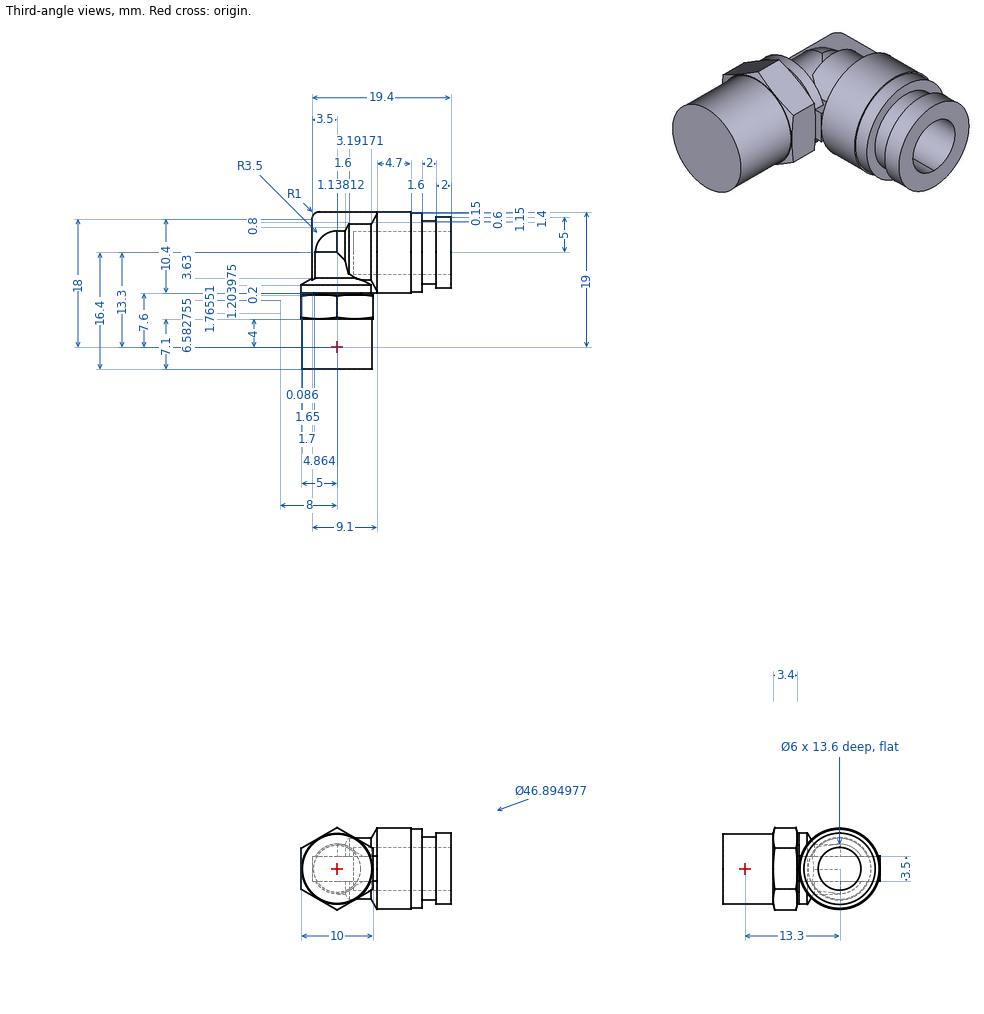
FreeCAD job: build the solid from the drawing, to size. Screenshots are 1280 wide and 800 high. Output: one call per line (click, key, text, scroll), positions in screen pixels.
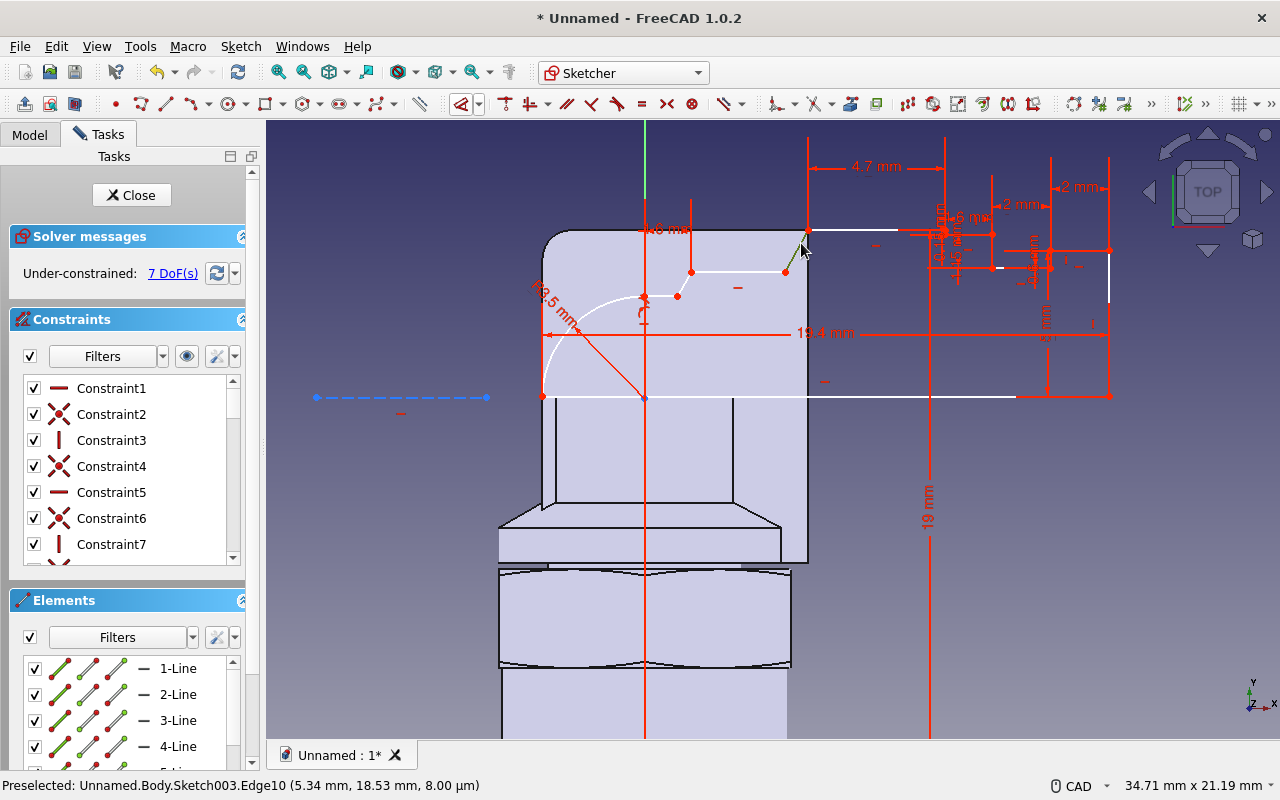
key(i)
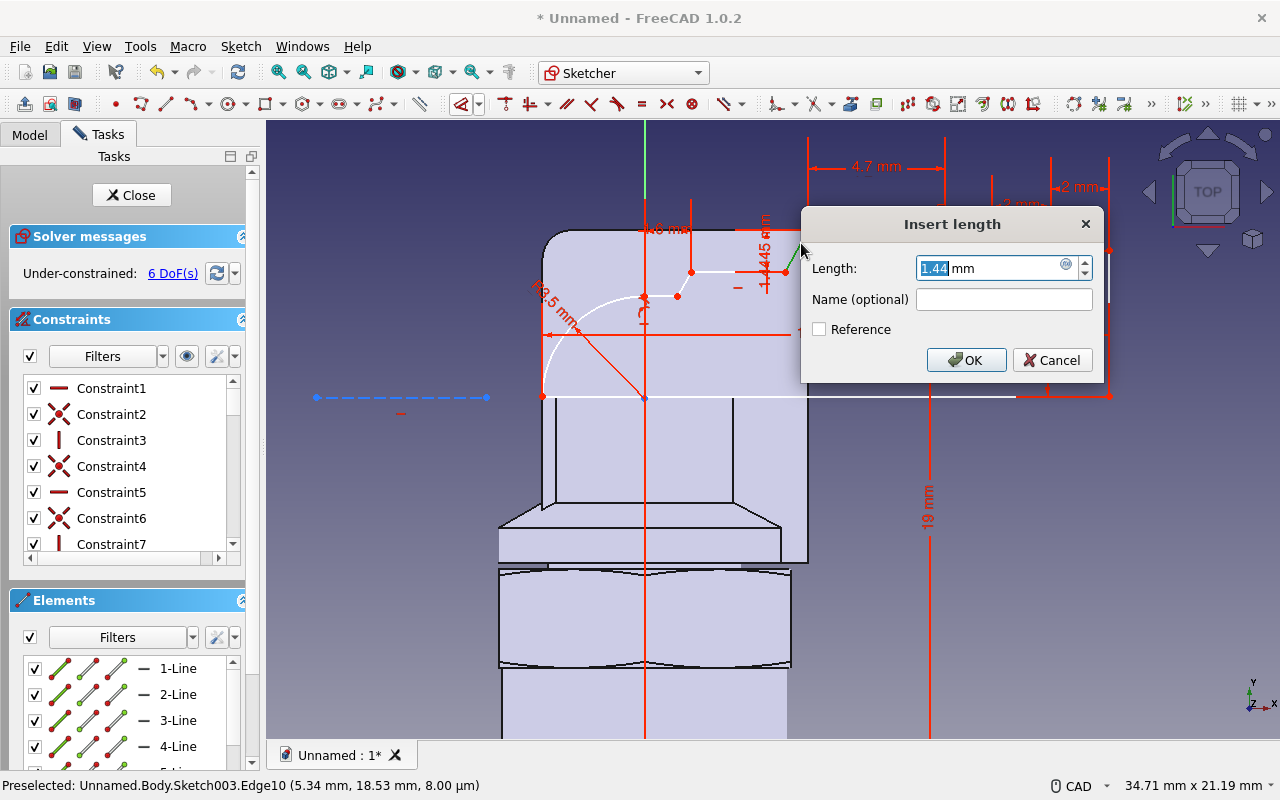
text(1.4)
key(Return)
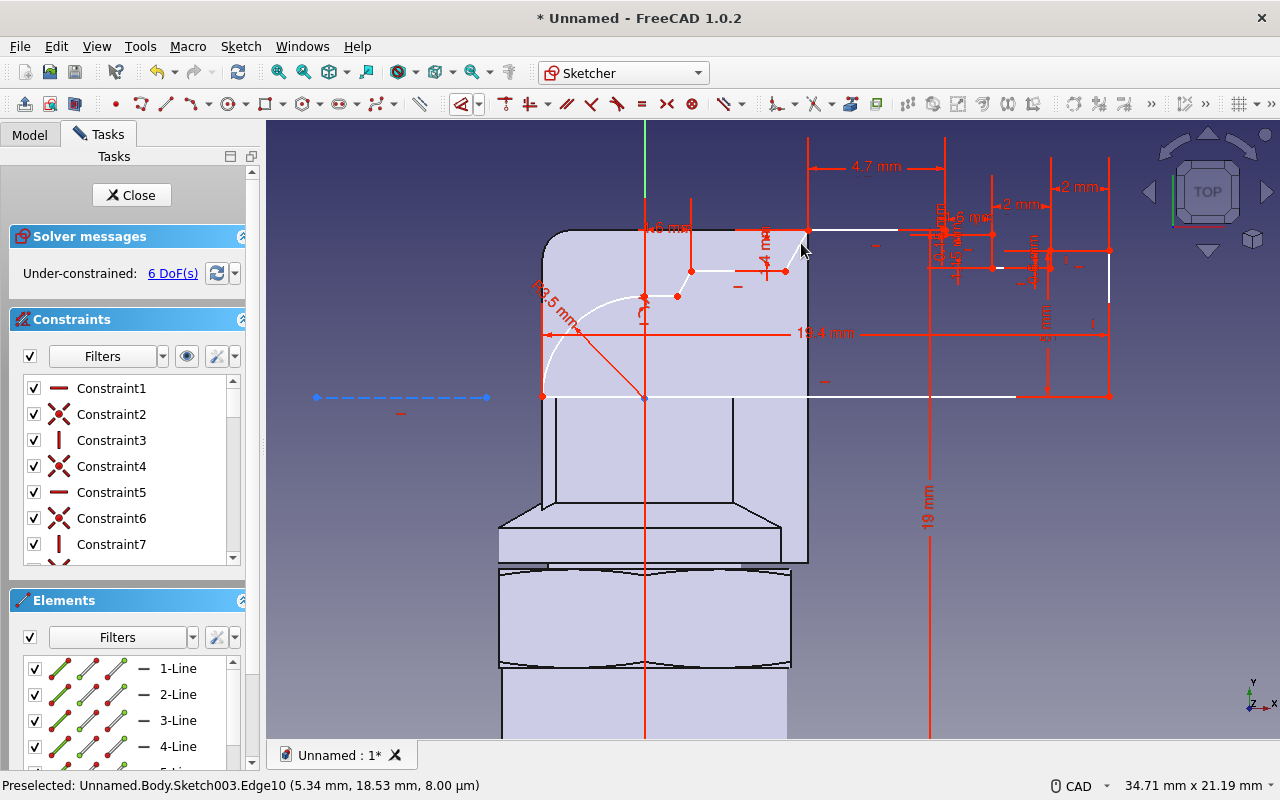
scroll(686, 281, up, 3)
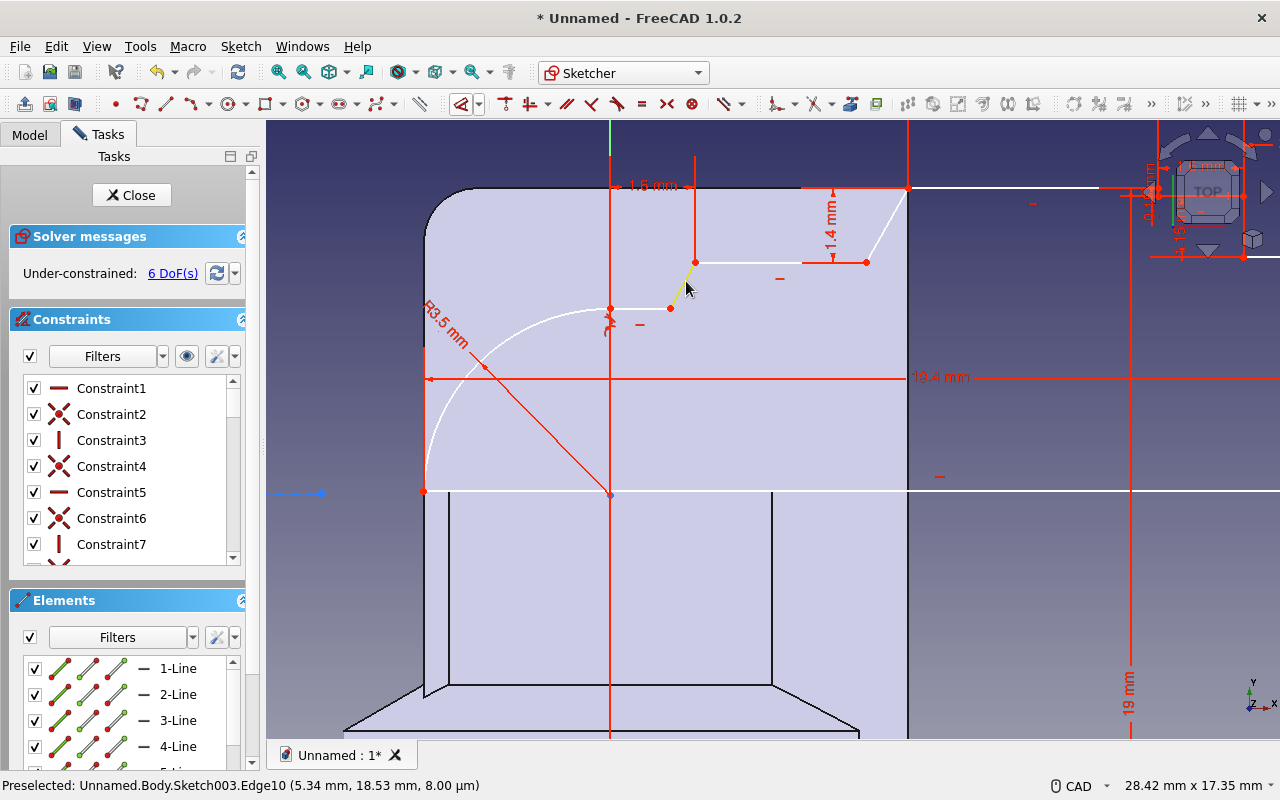
click(685, 281)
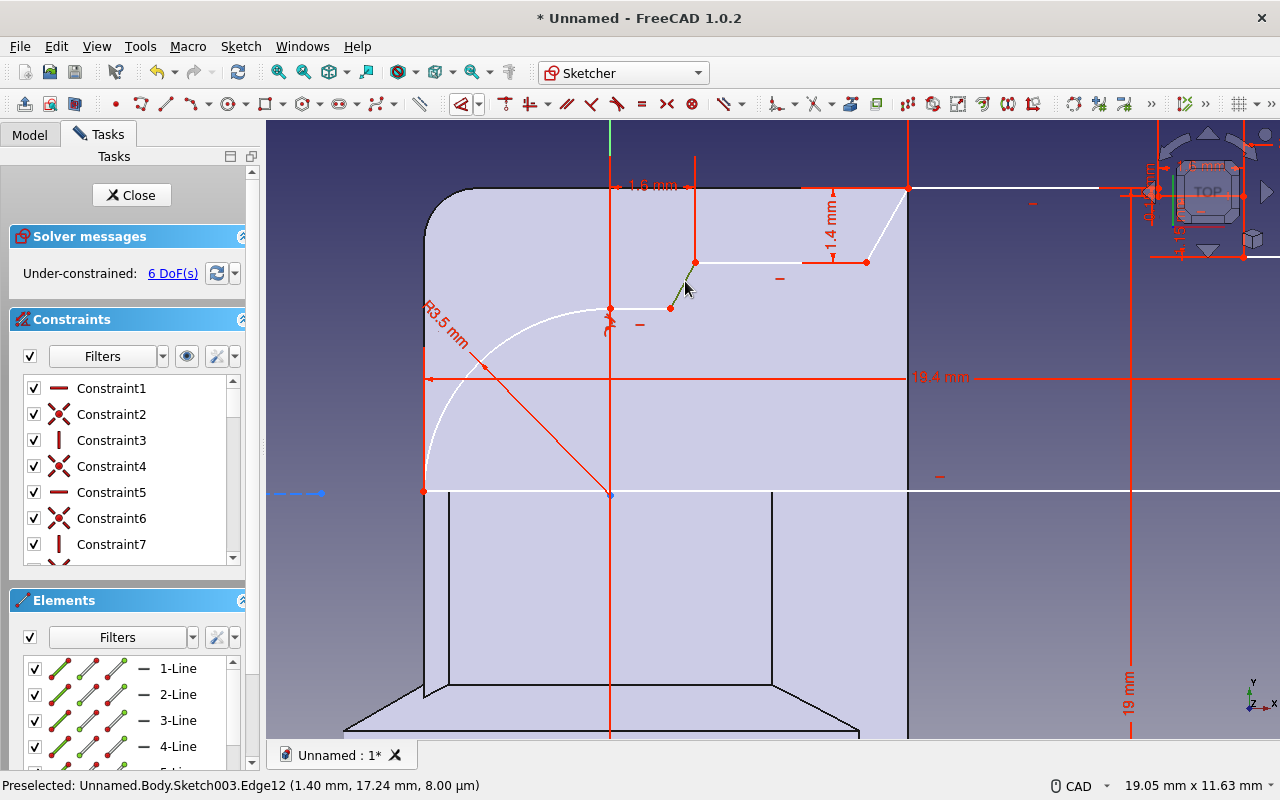
click(478, 104)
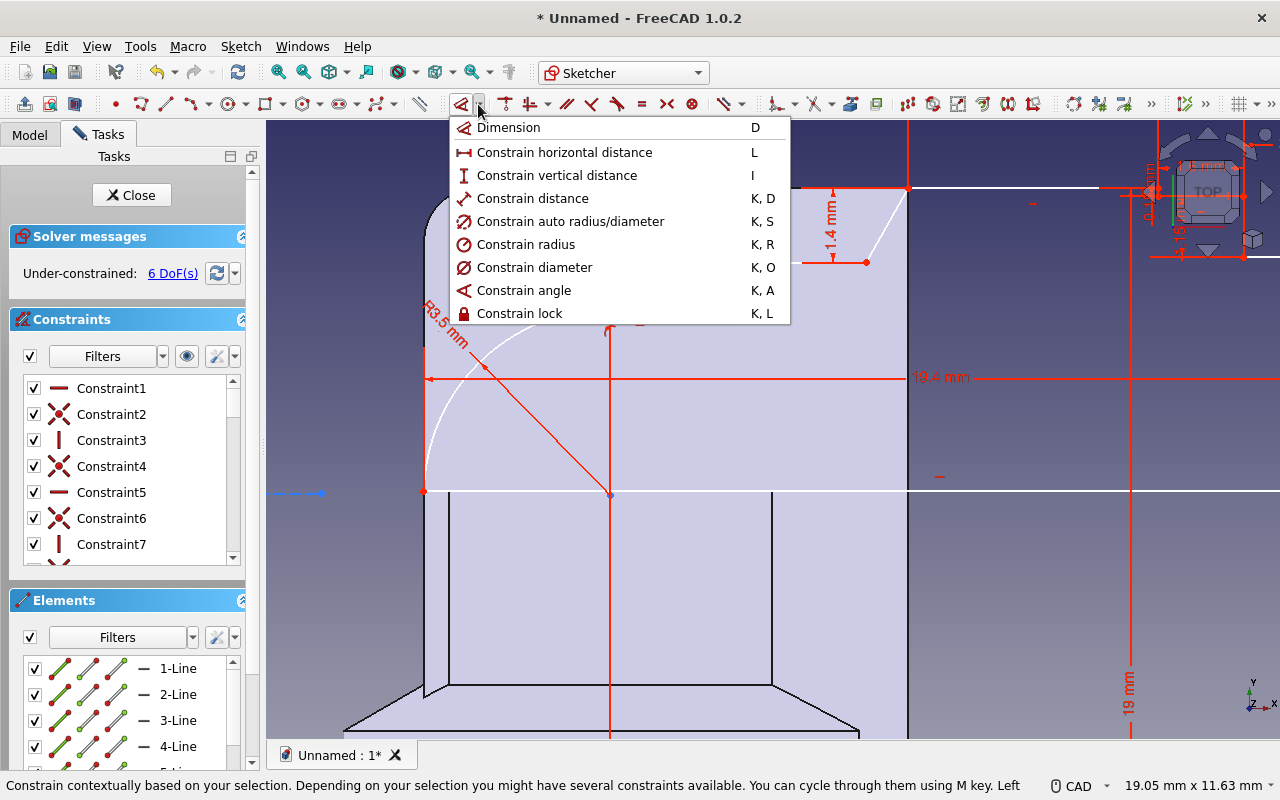
click(620, 176)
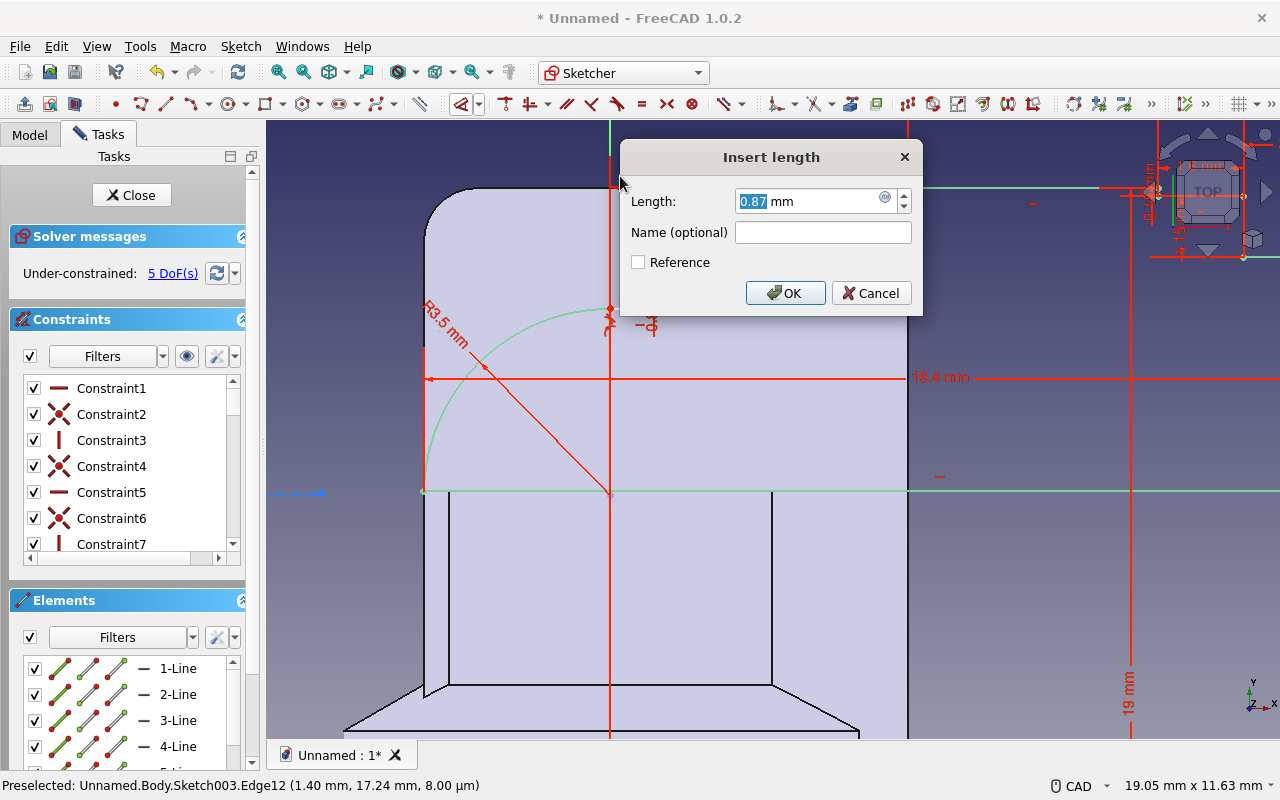
text(0.8)
key(Return)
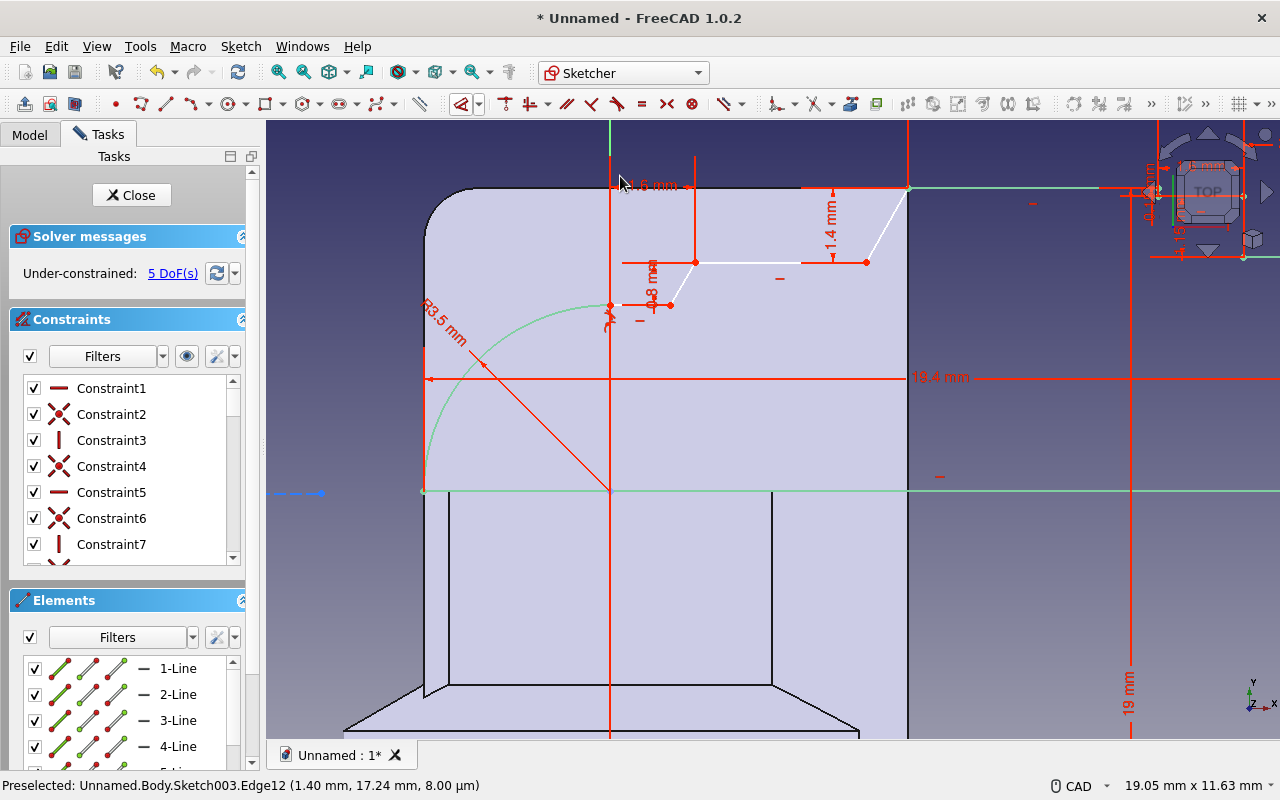
click(321, 494)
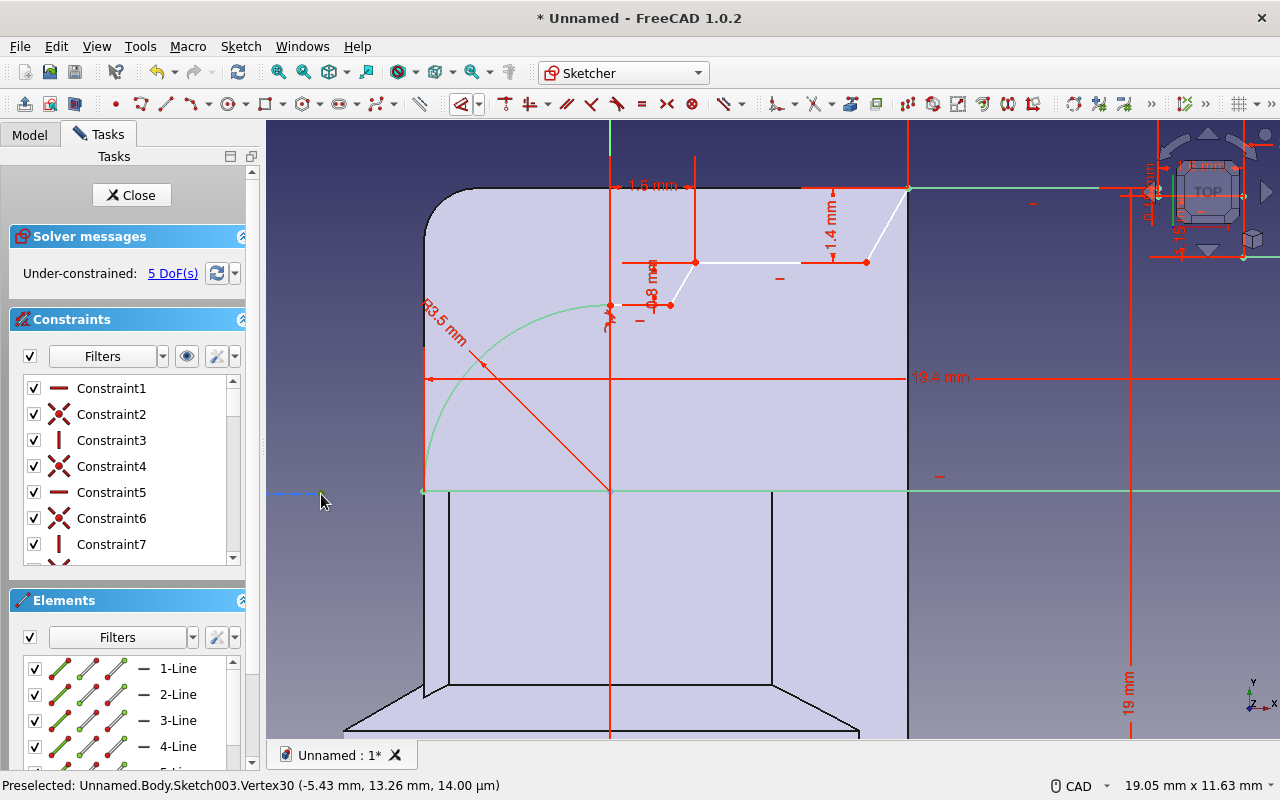
key(i)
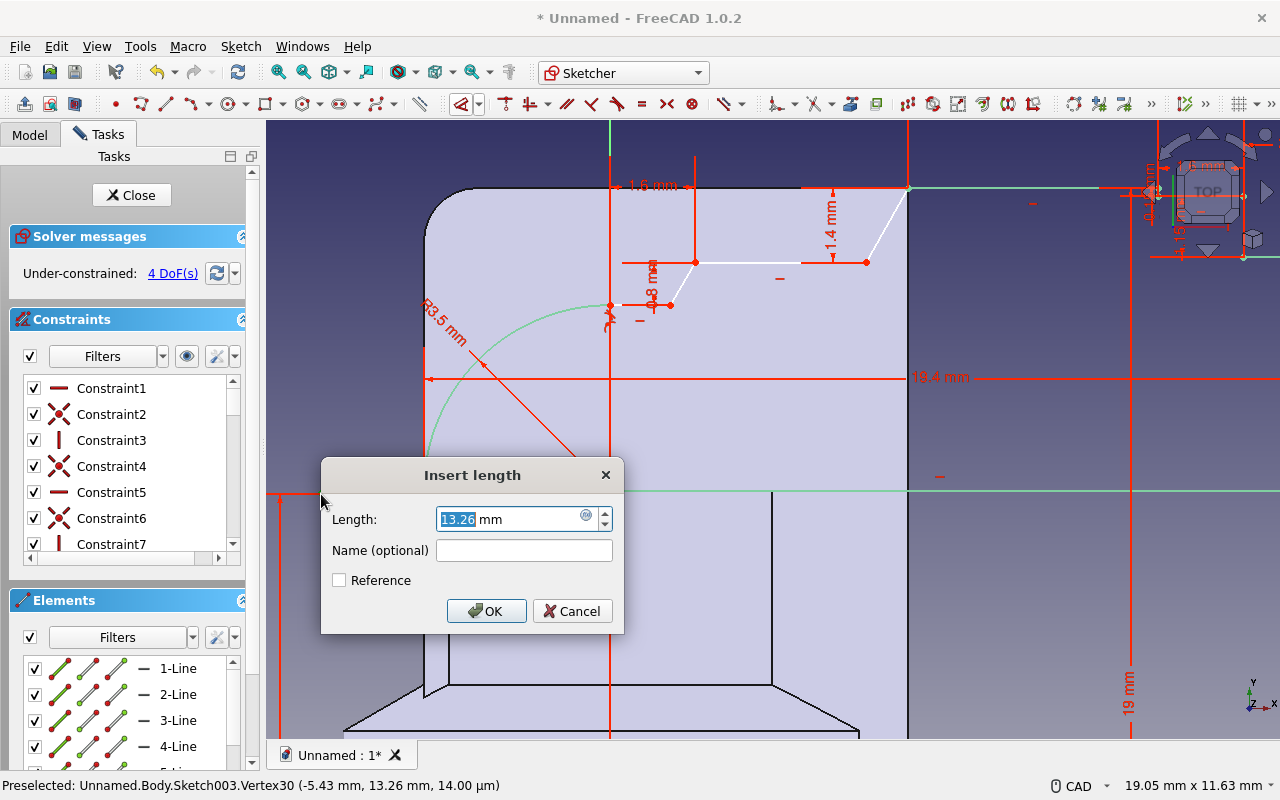
text(13.3)
key(Return)